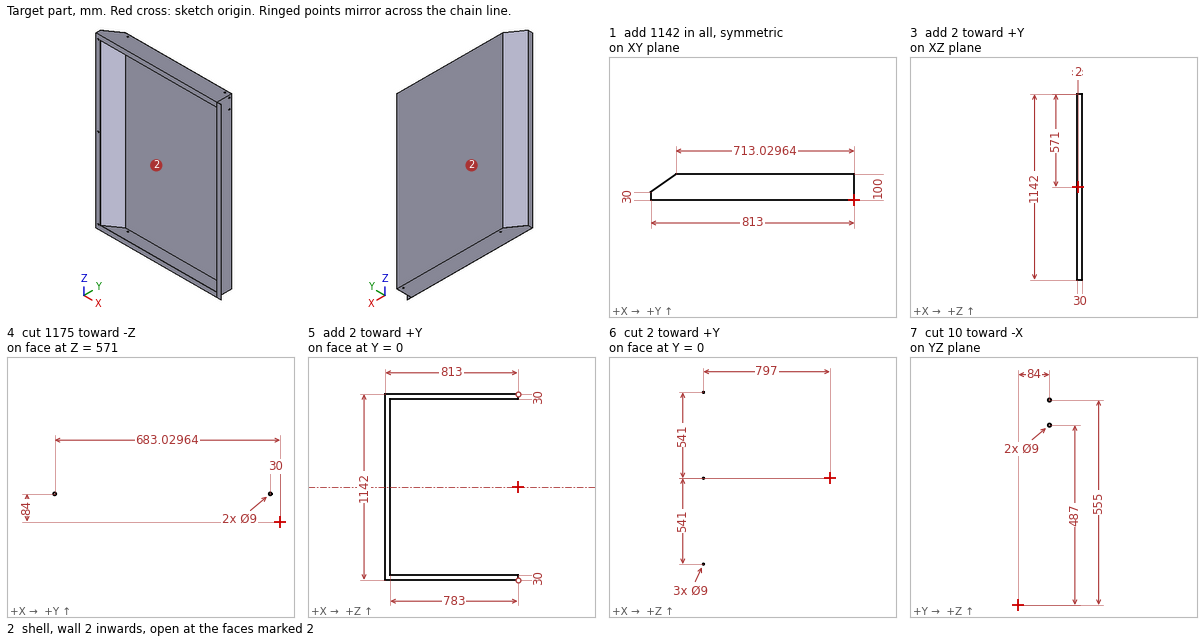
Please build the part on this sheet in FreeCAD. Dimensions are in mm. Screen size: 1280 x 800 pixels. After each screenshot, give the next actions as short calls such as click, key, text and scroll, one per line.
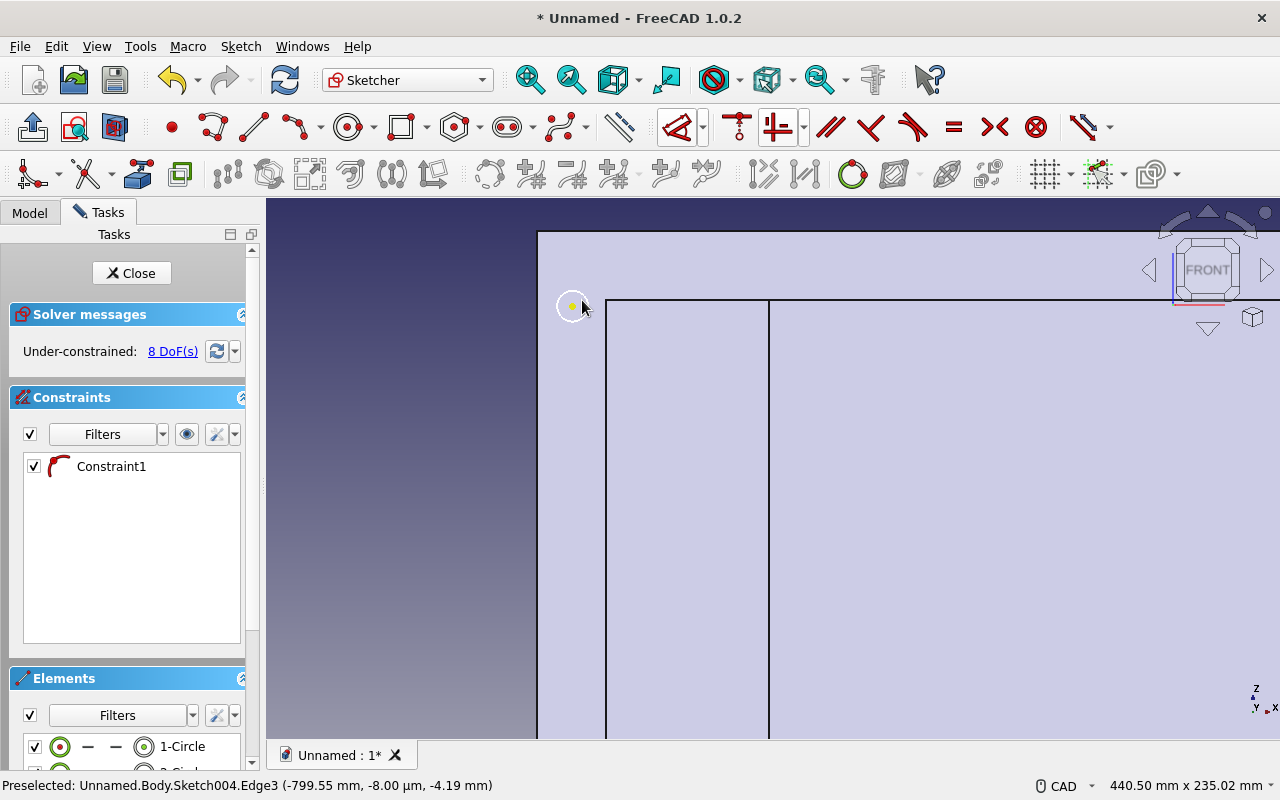
click(584, 295)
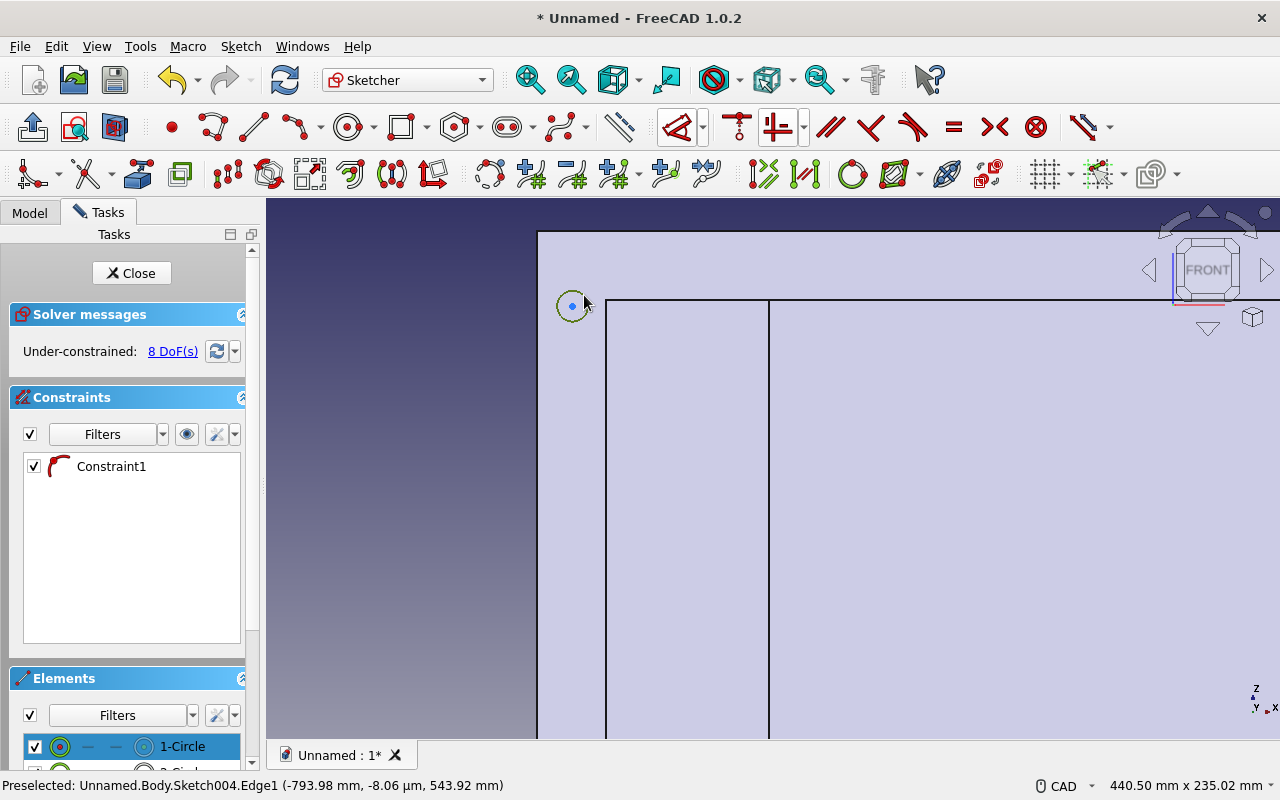
scroll(582, 300, down, 10)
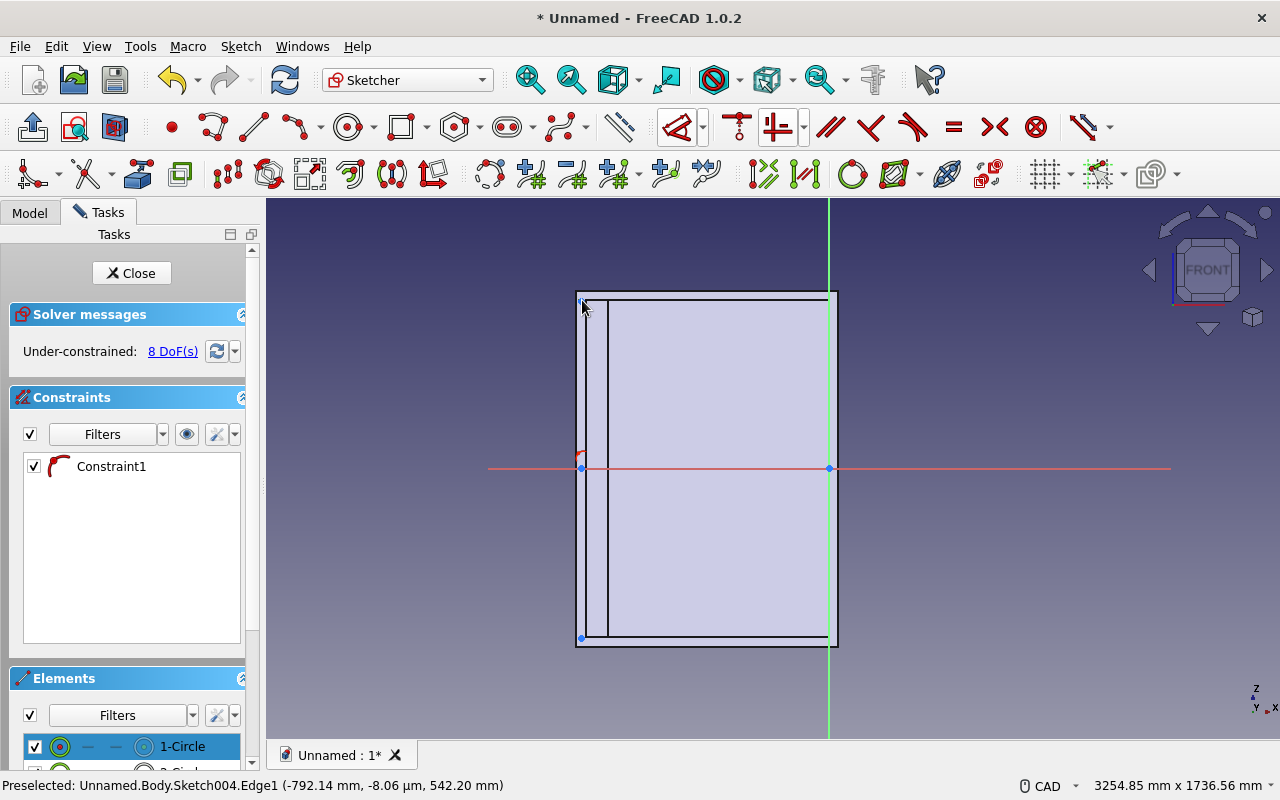
scroll(582, 637, up, 10)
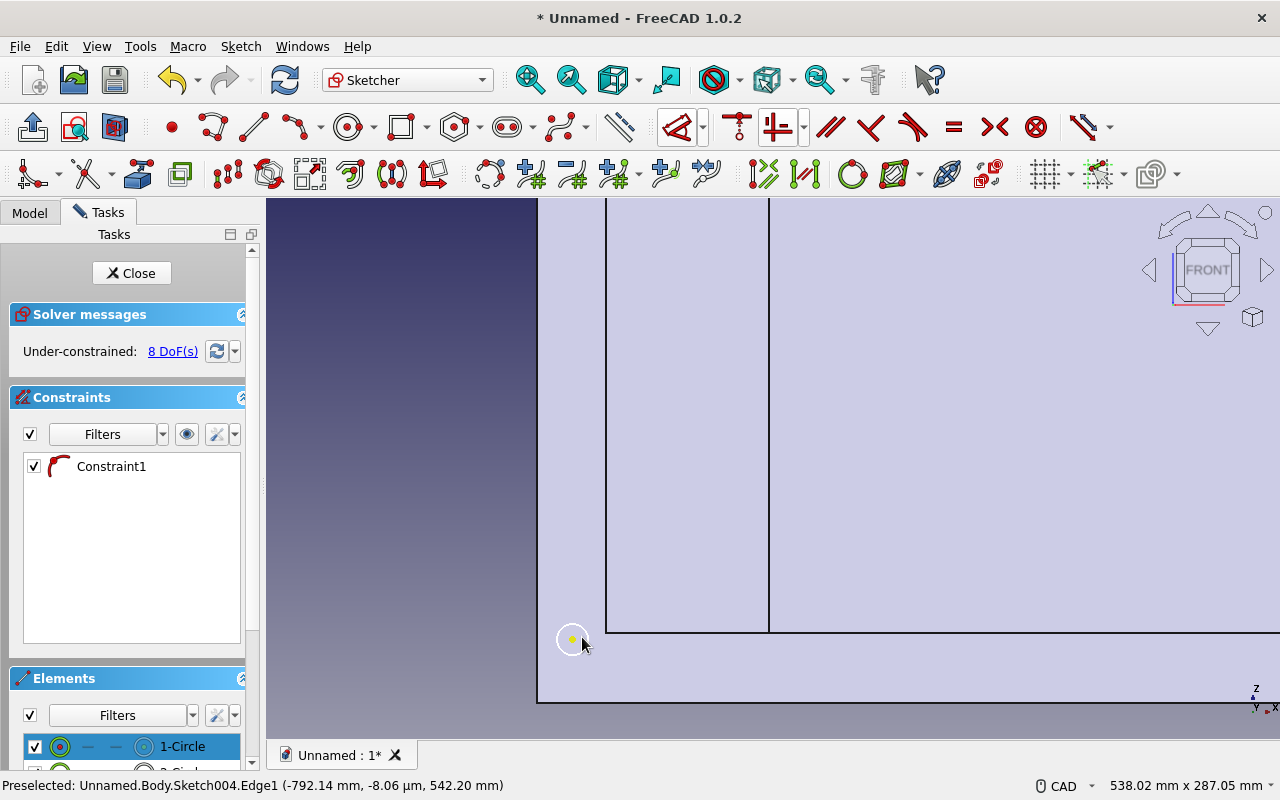
click(584, 629)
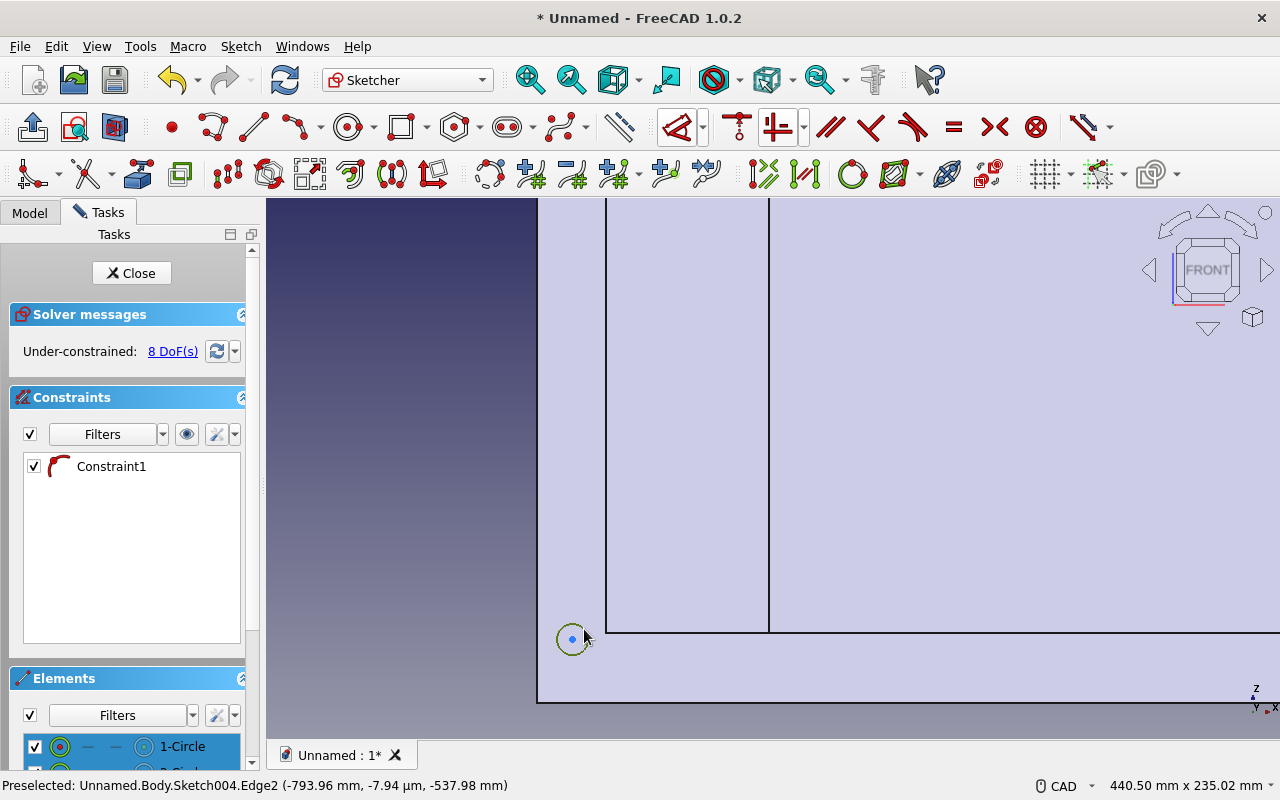
scroll(582, 638, down, 10)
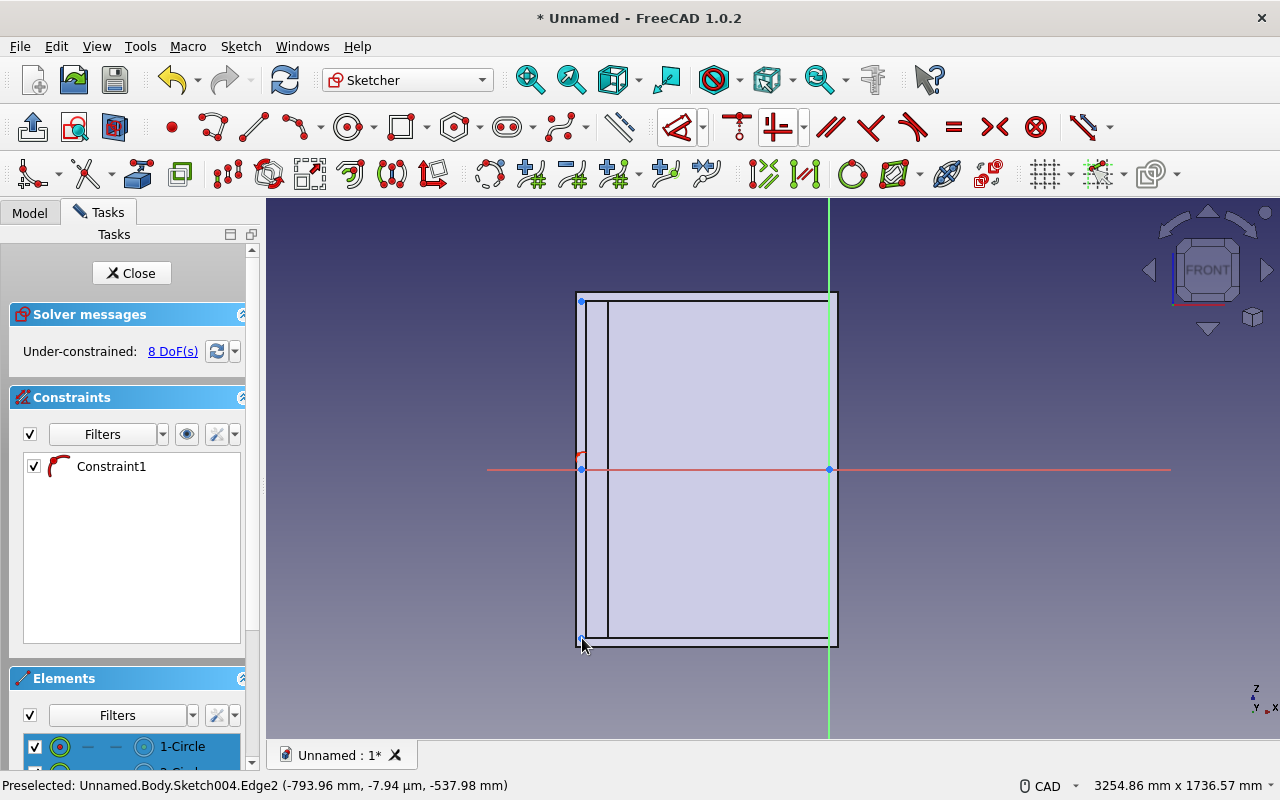
scroll(581, 468, up, 12)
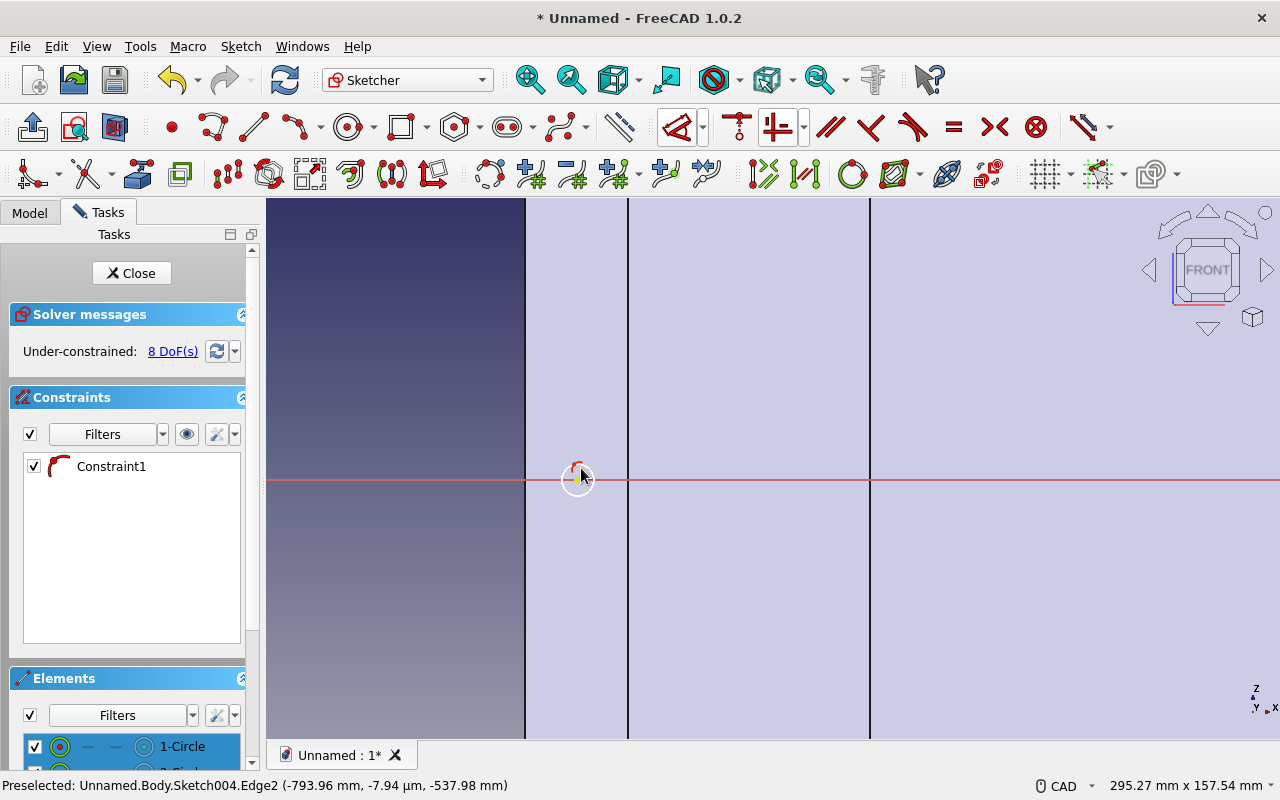
click(562, 480)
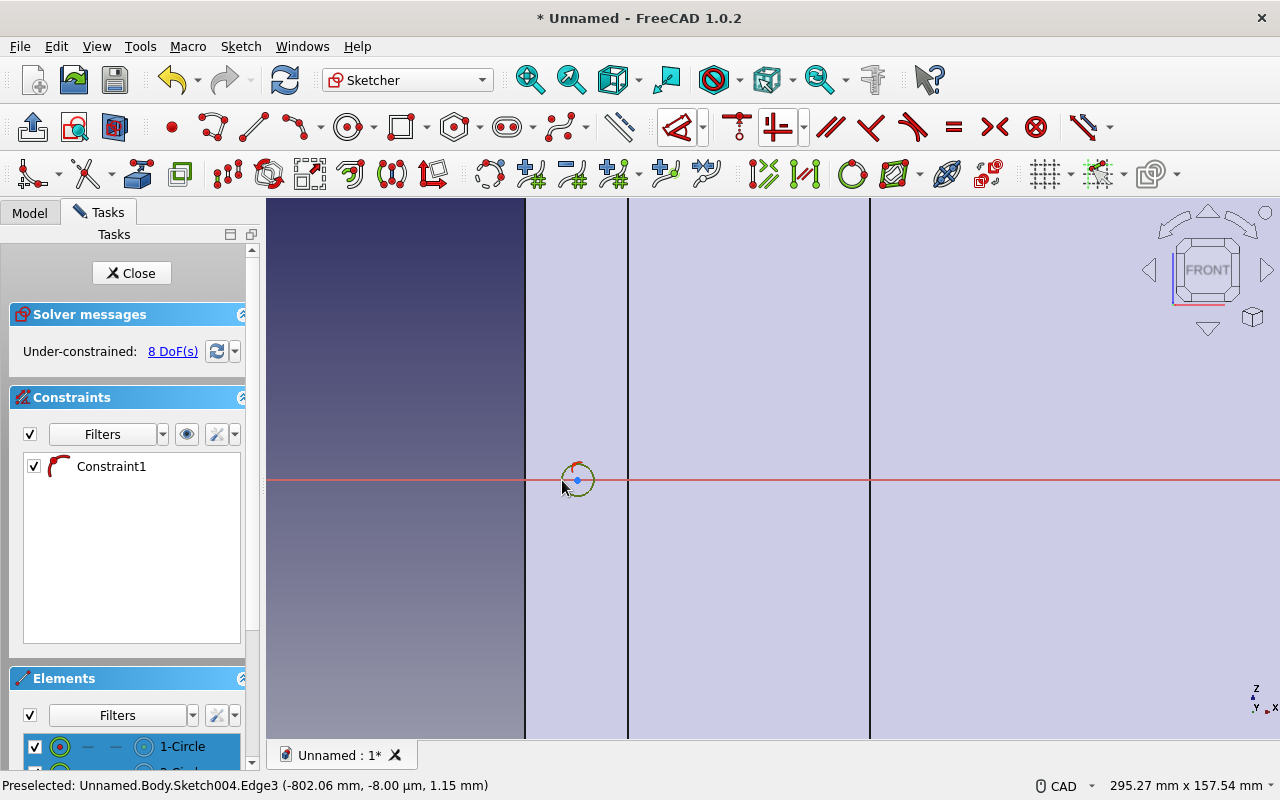
click(954, 128)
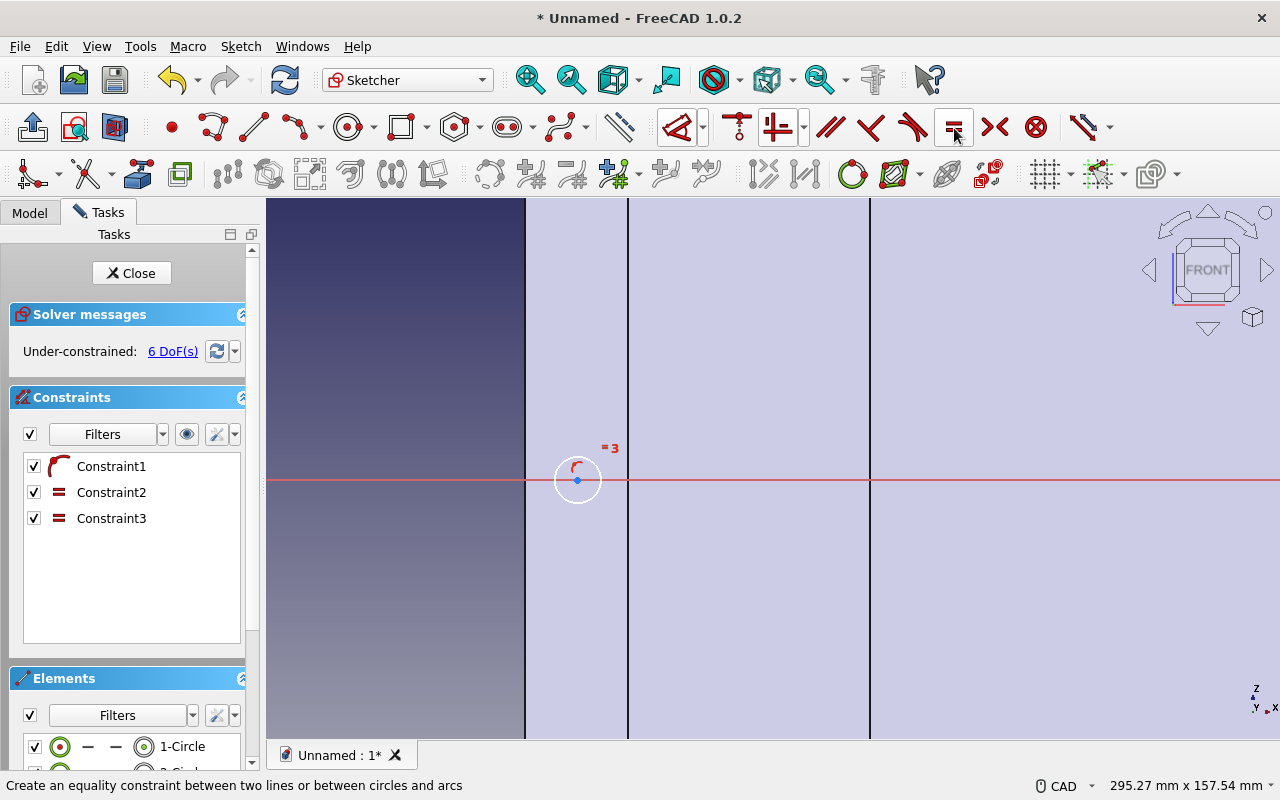
scroll(581, 467, down, 12)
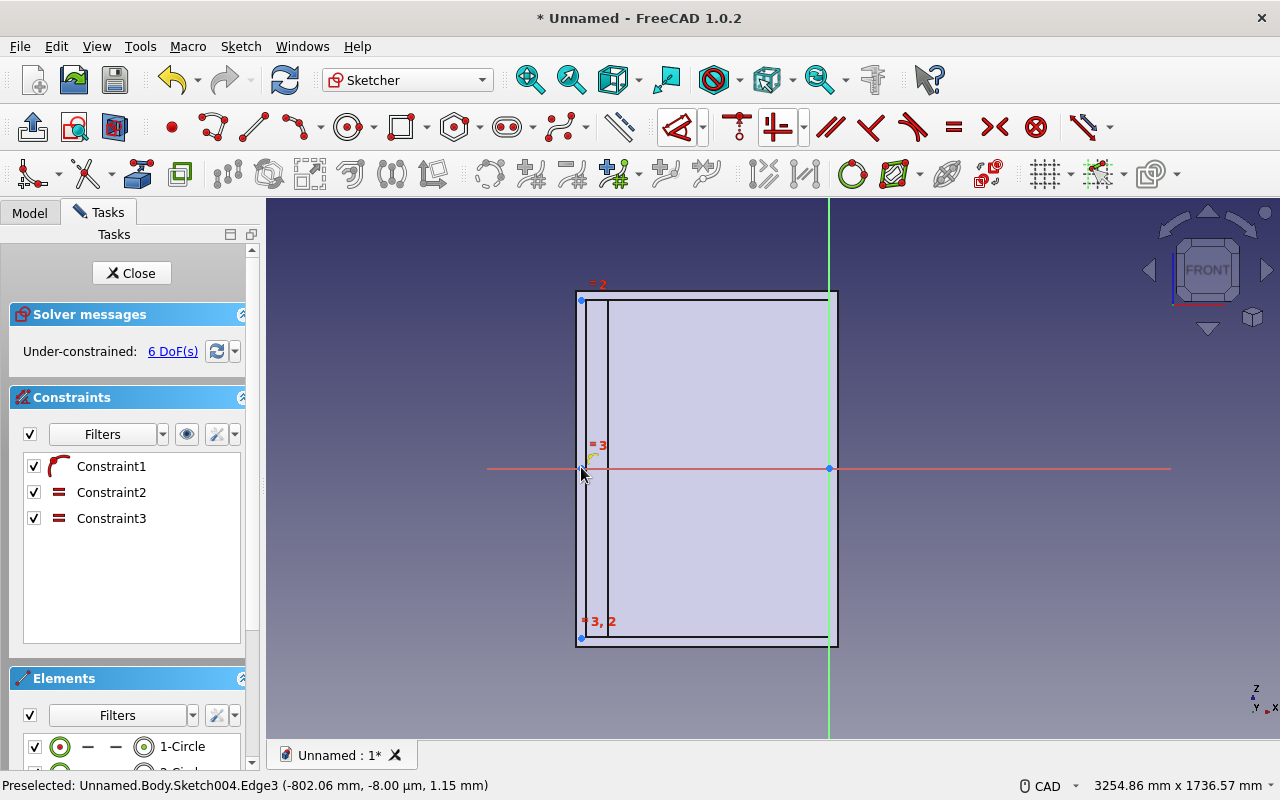
click(581, 301)